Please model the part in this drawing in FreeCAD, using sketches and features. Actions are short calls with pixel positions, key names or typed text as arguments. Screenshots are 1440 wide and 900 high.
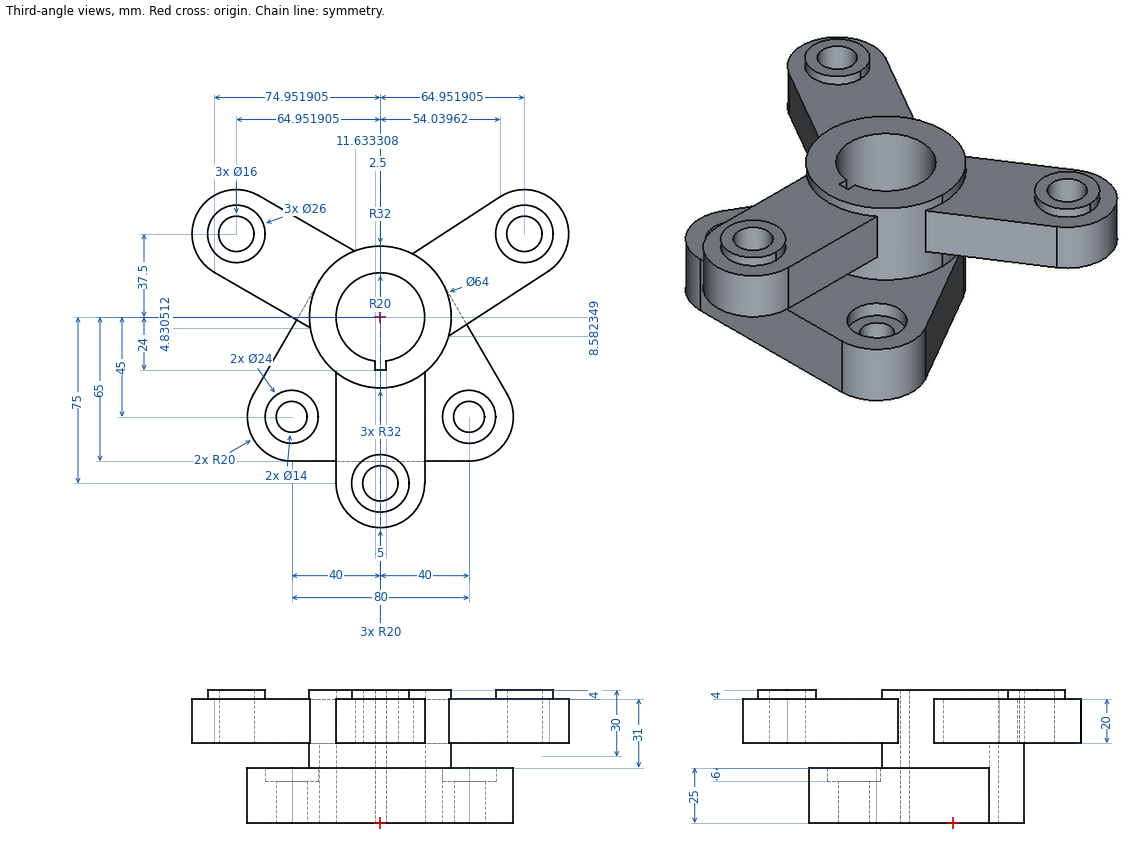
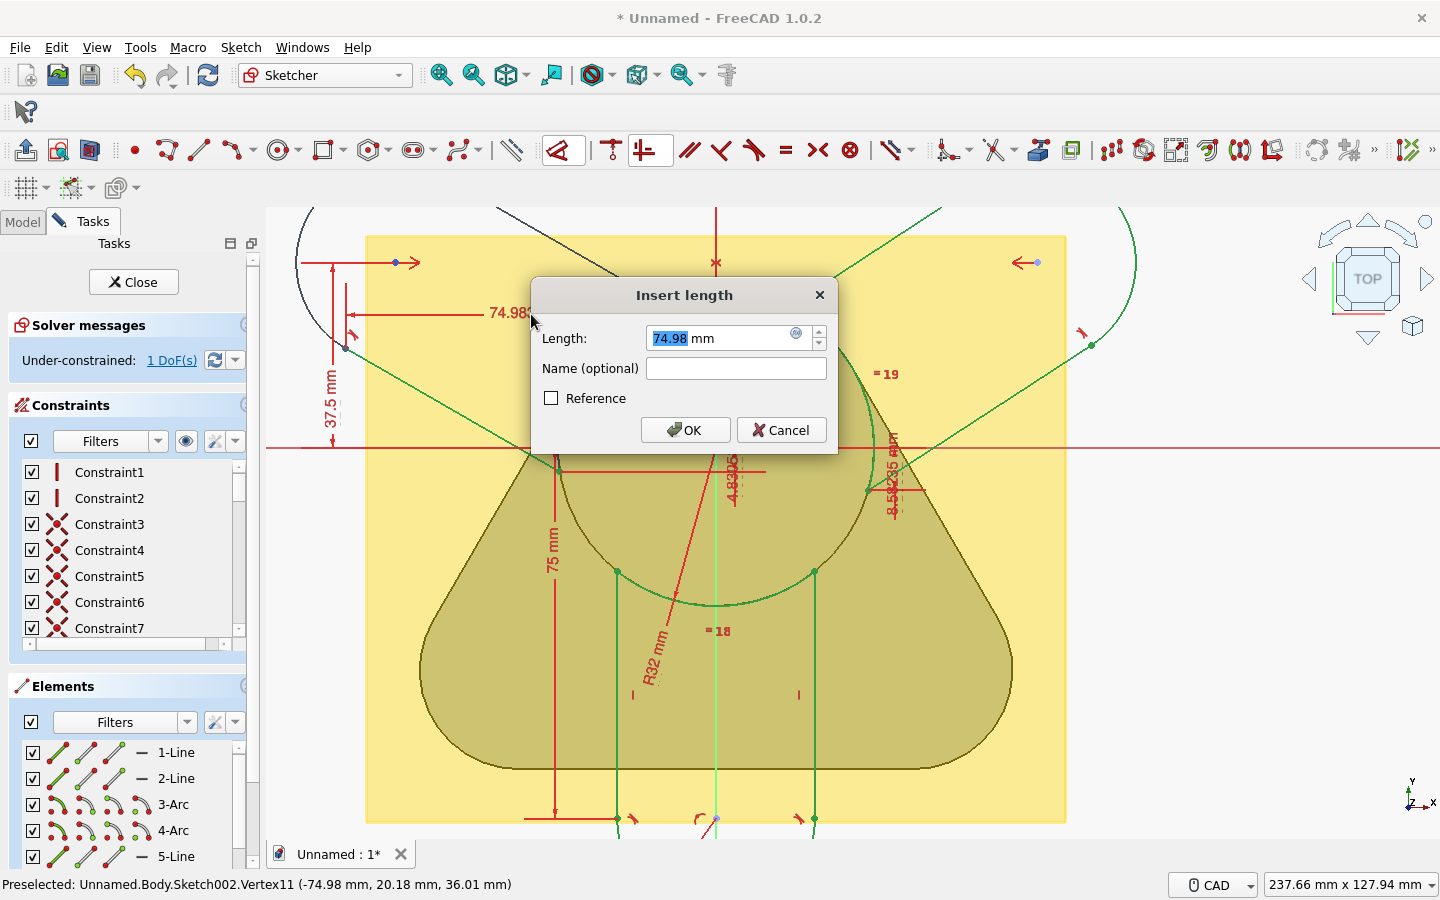
text(74.951905)
key(Return)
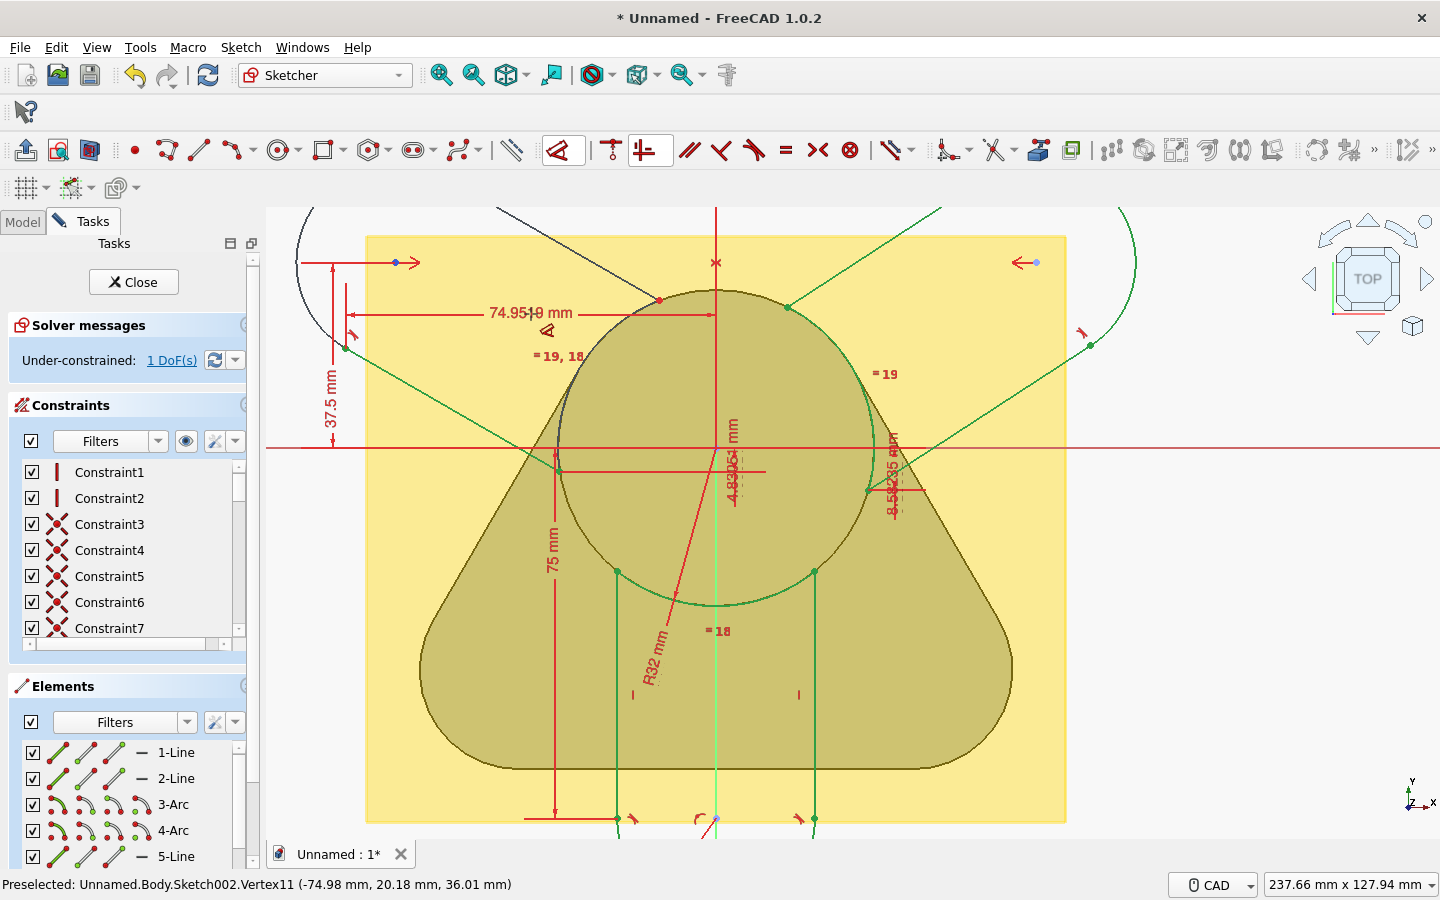
click(659, 301)
click(688, 267)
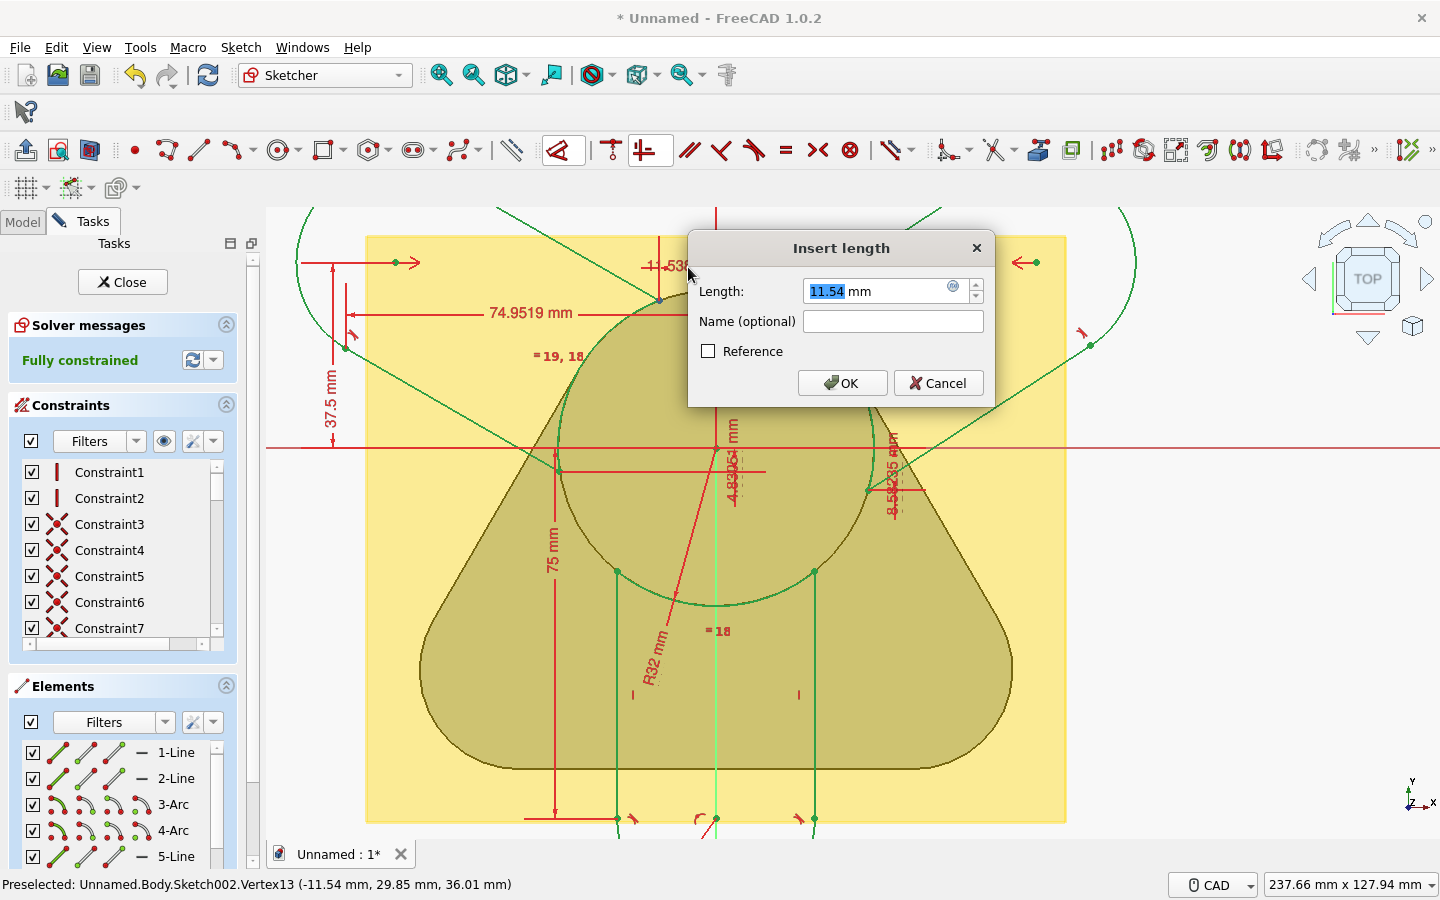
text(11.633308)
key(Return)
key(Escape)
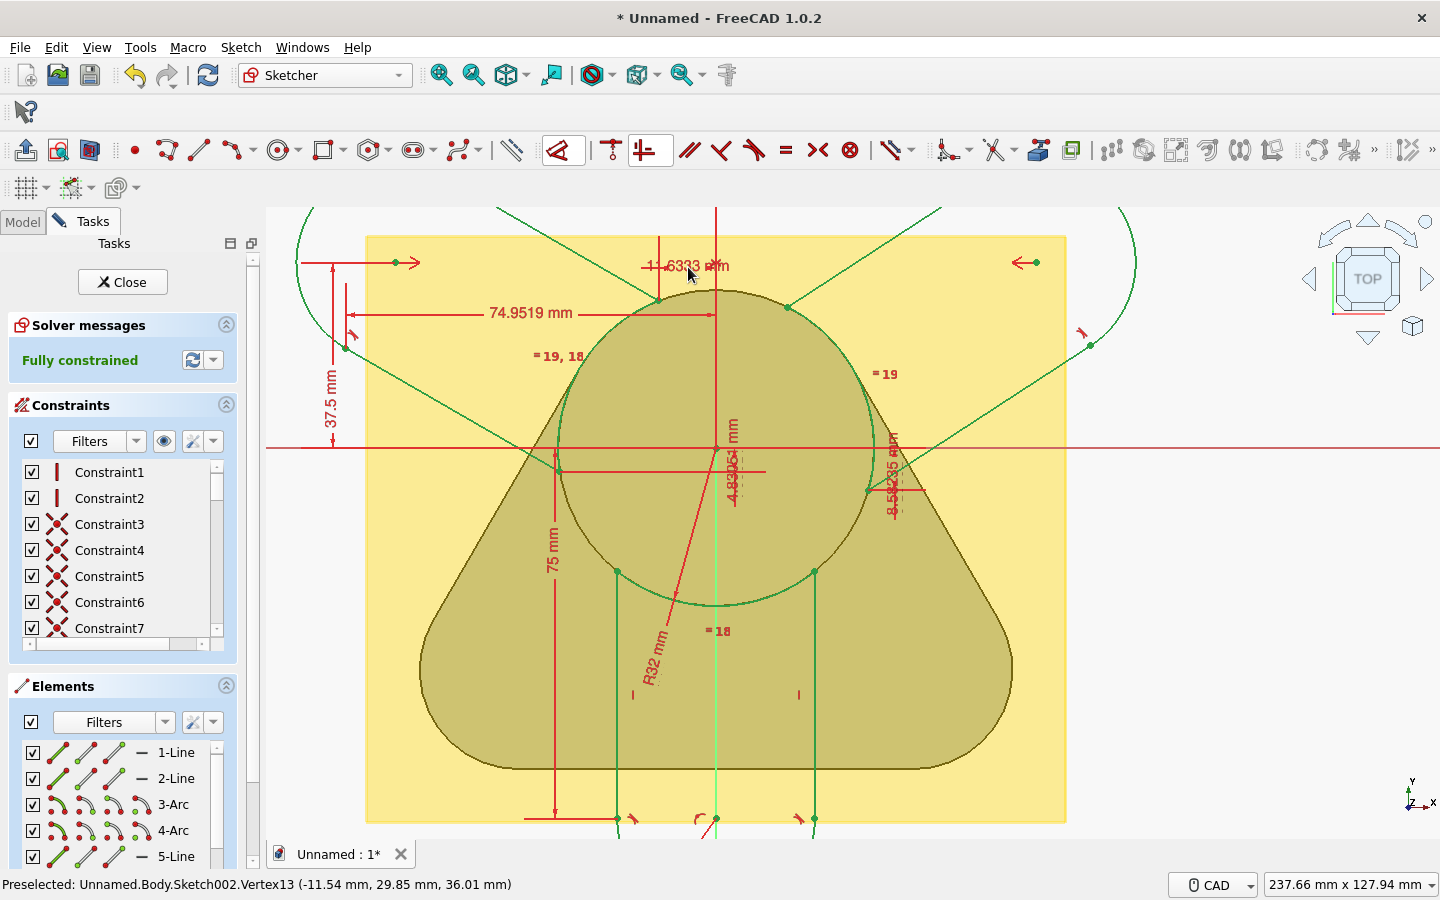
click(123, 282)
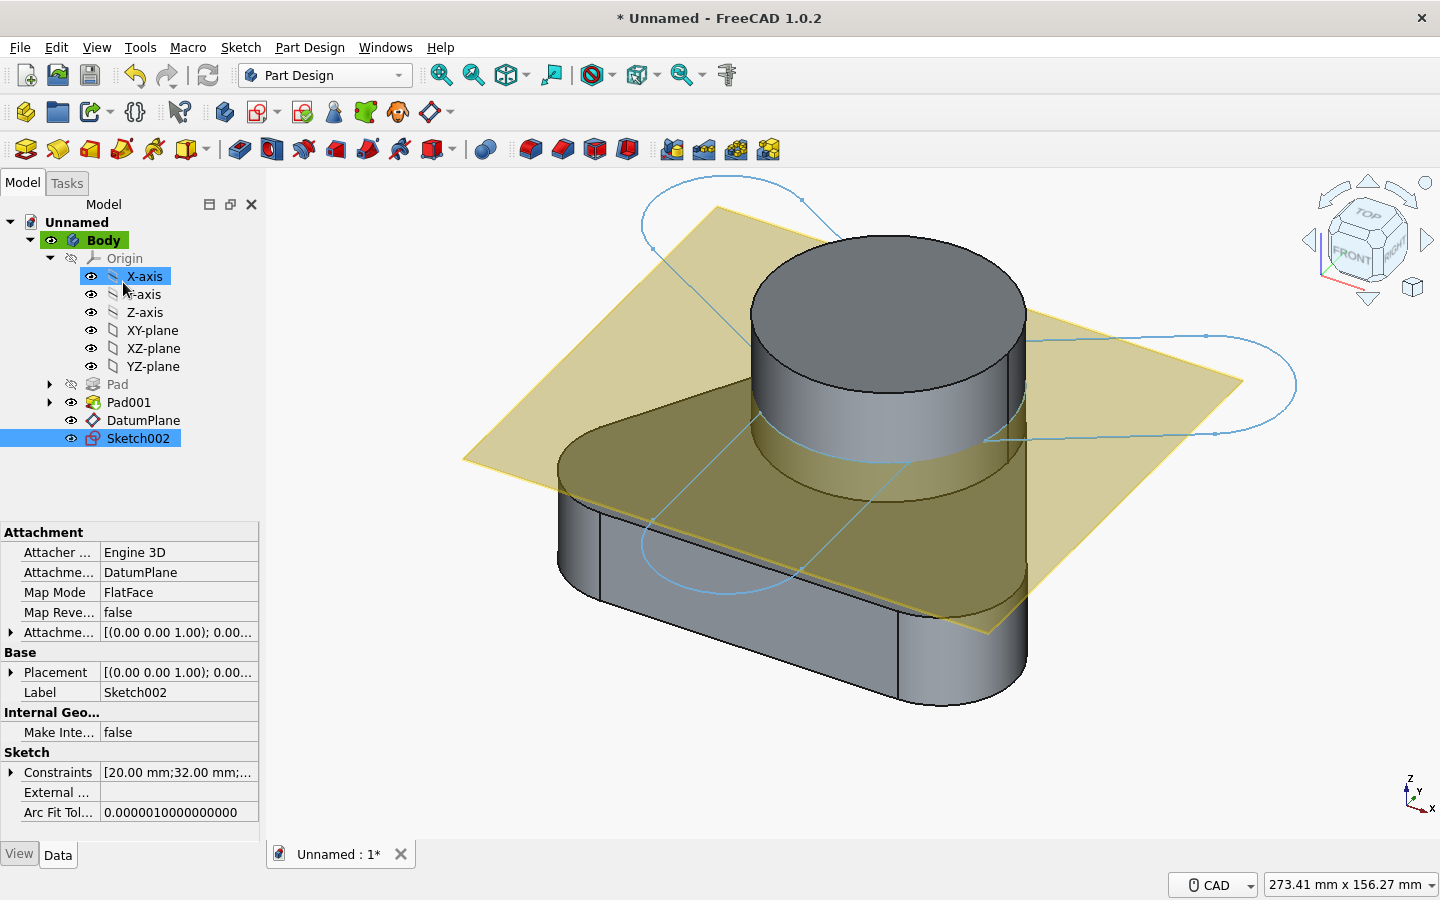
click(26, 150)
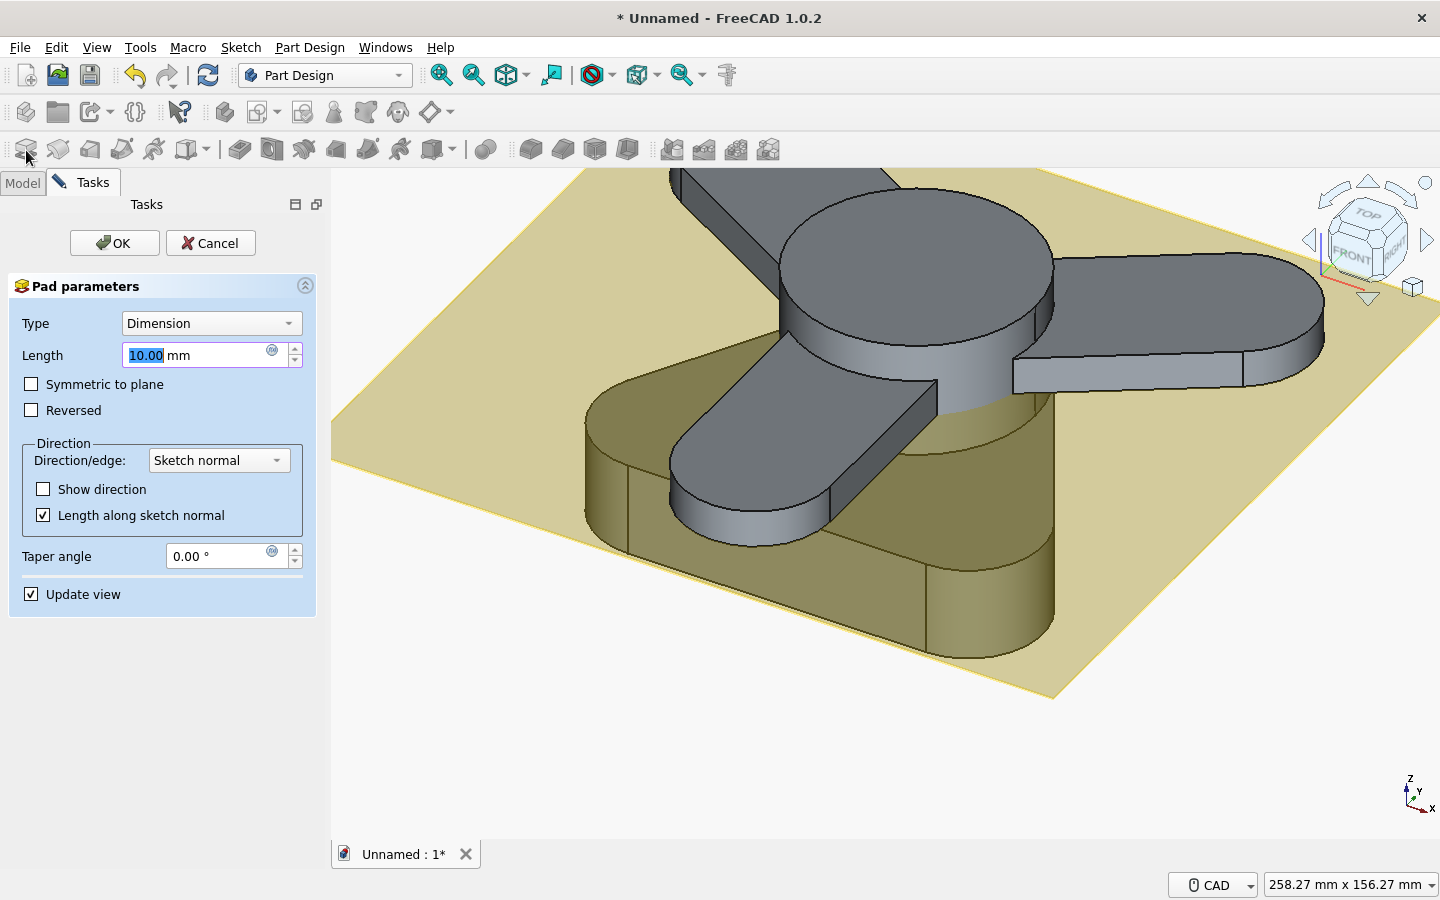
text(20)
key(Tab)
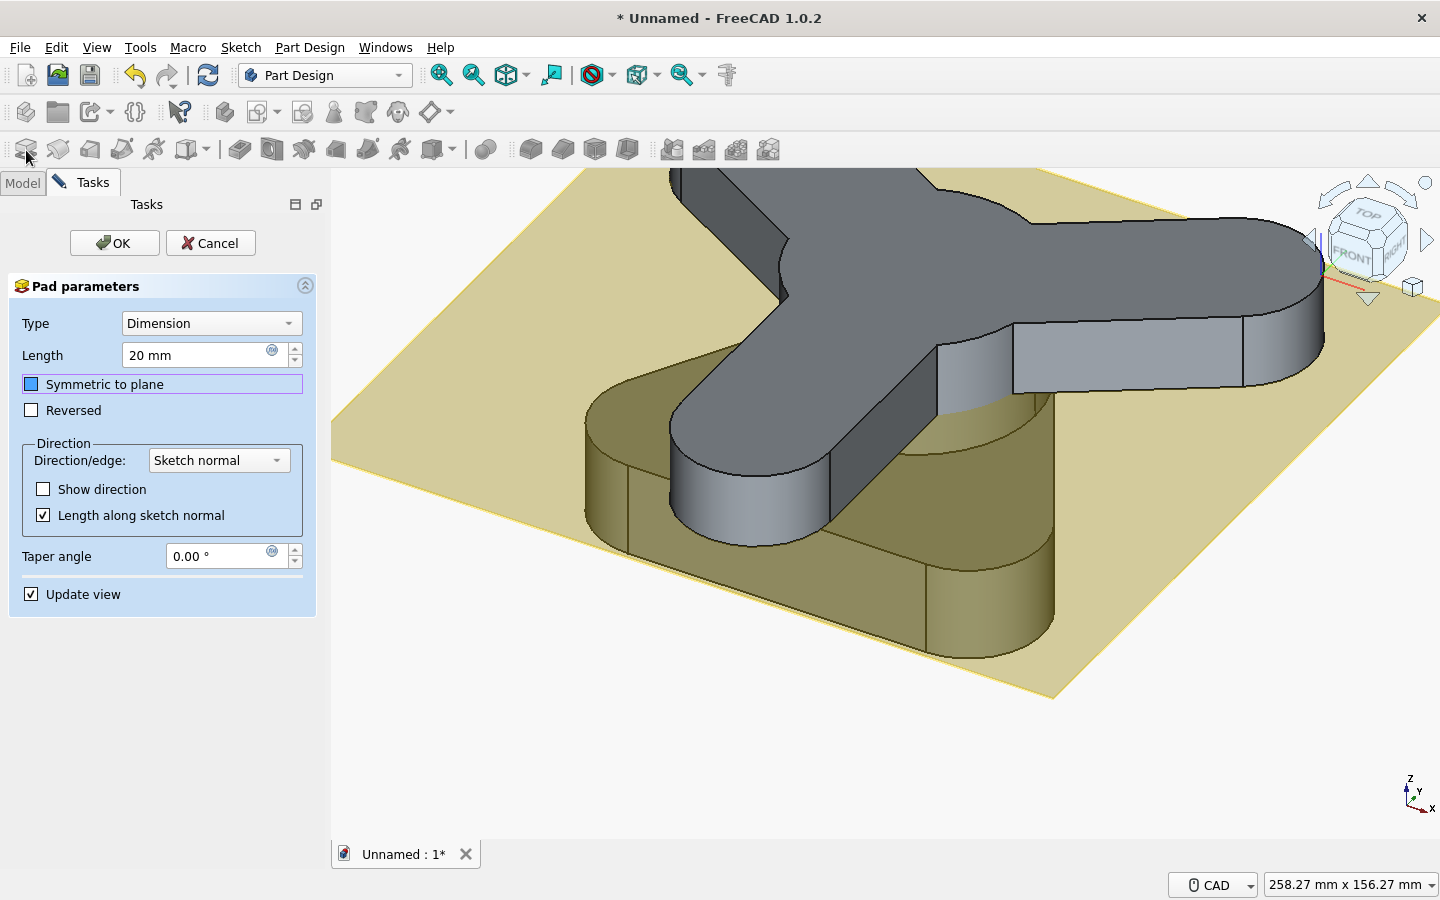
click(115, 243)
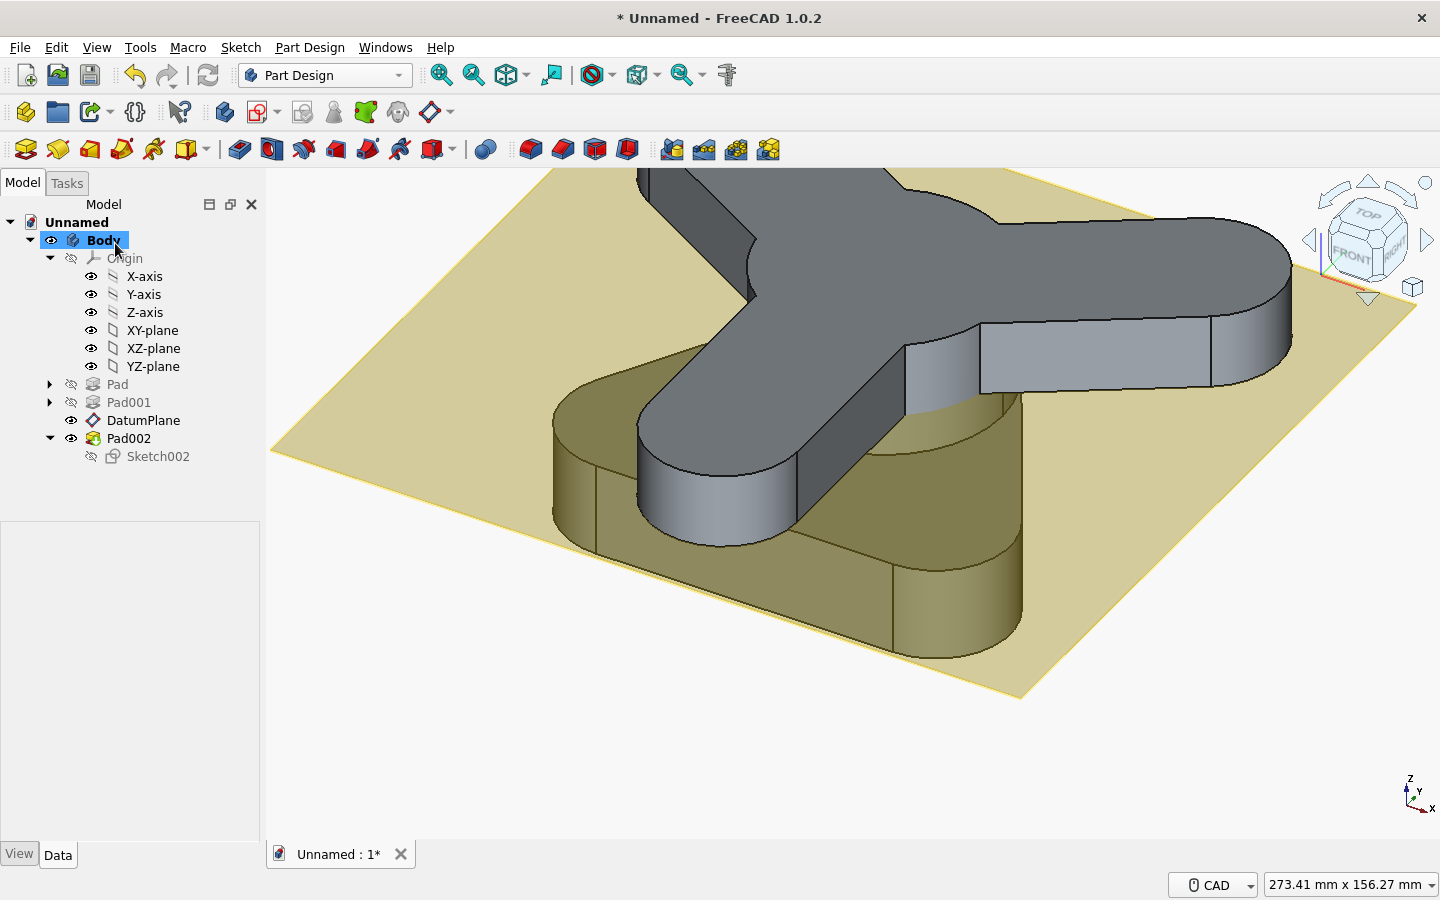
click(116, 420)
key(space)